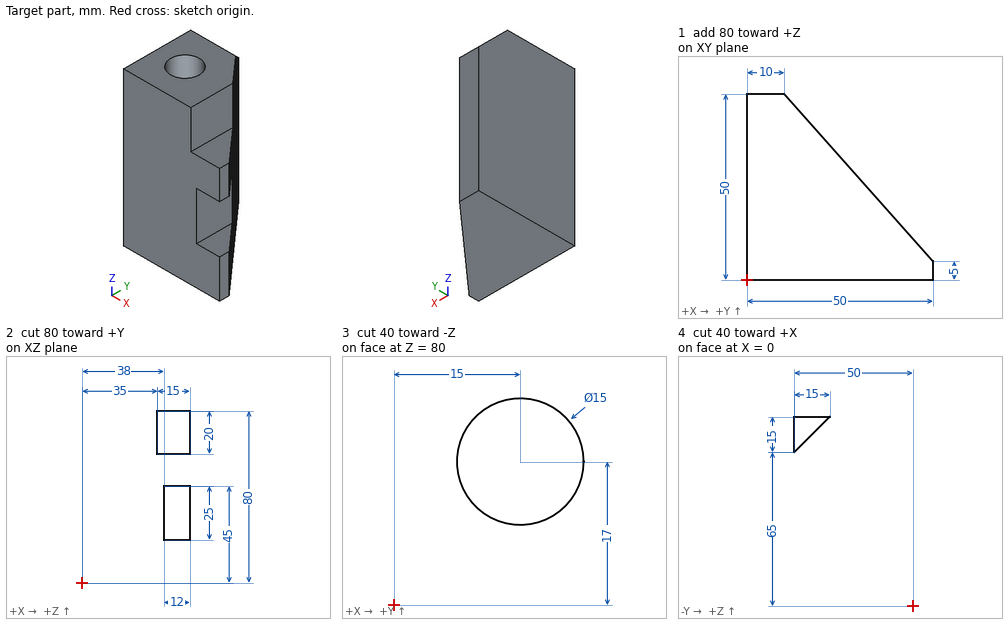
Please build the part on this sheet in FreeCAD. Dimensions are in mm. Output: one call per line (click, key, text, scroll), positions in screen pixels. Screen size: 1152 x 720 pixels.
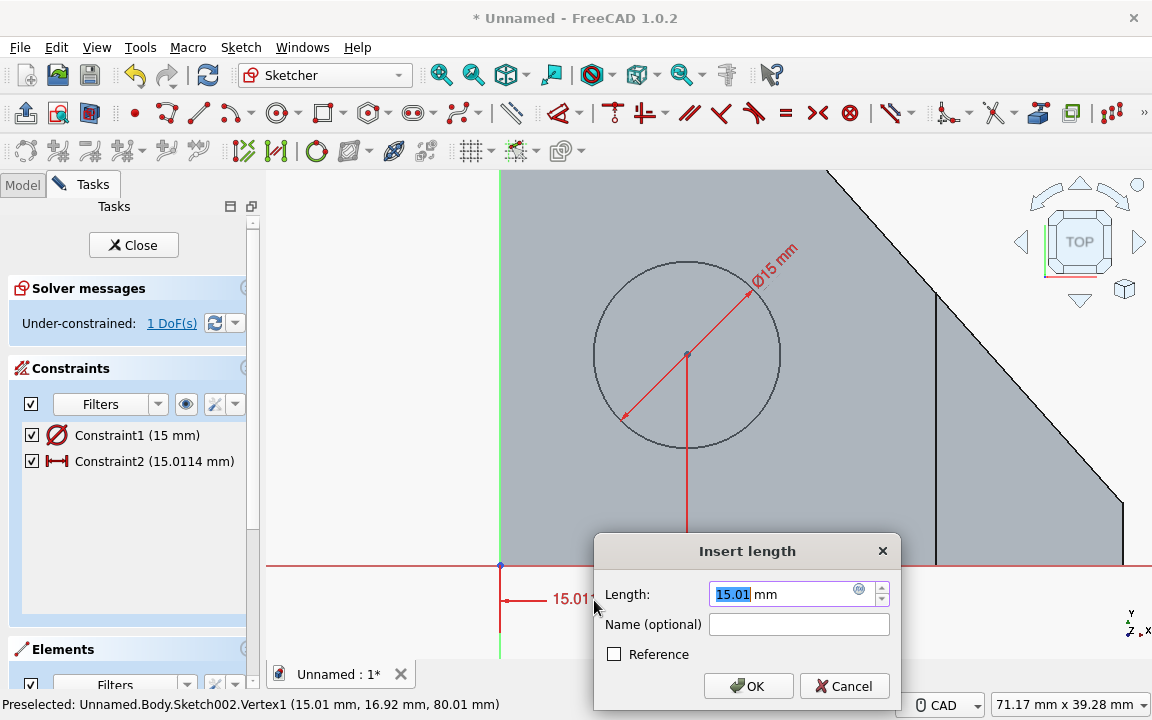
text(15)
key(Return)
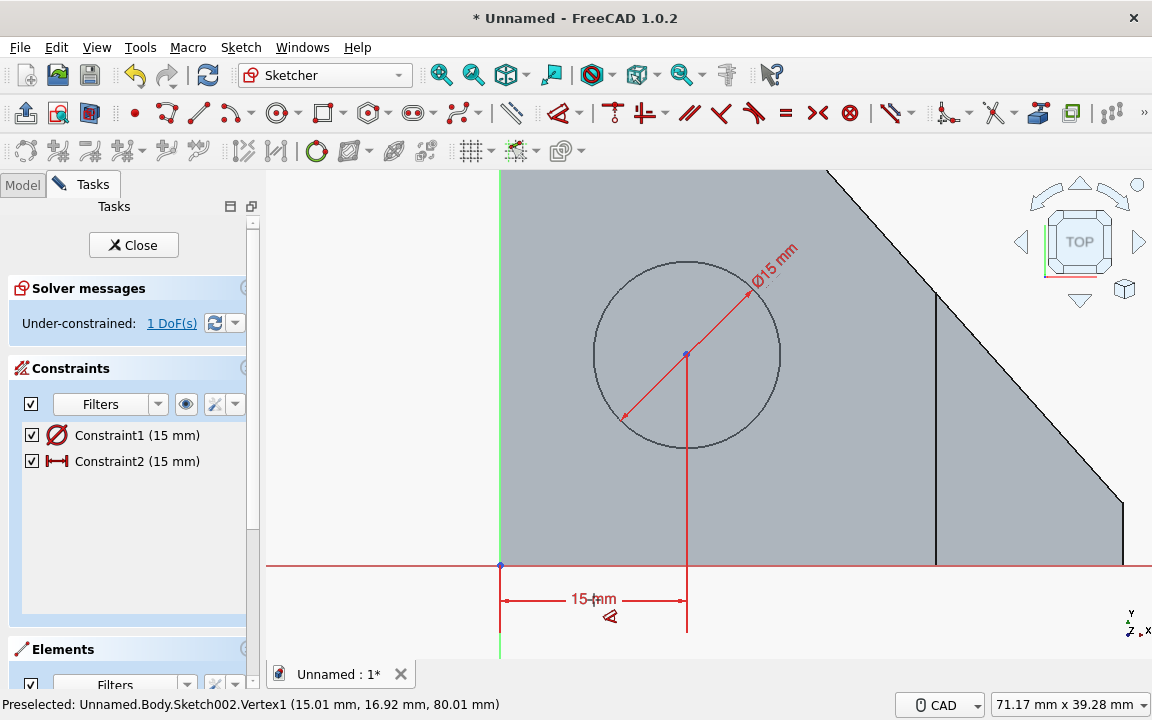
click(687, 355)
click(466, 460)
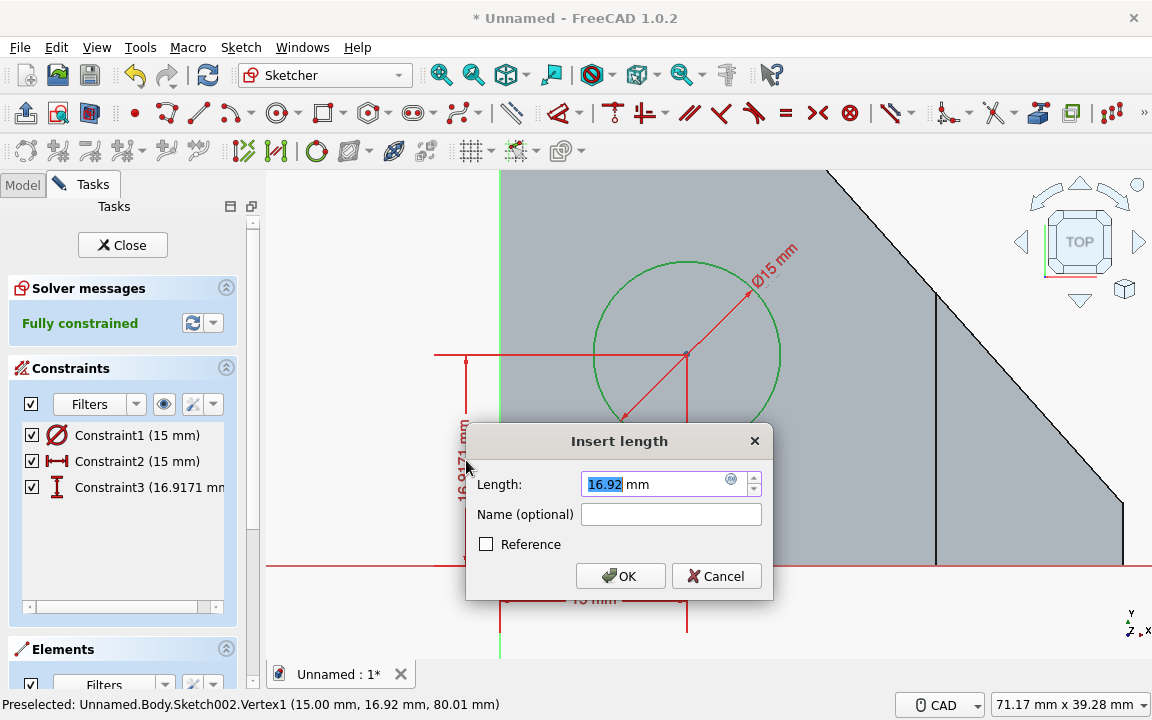
text(17)
key(Return)
key(Escape)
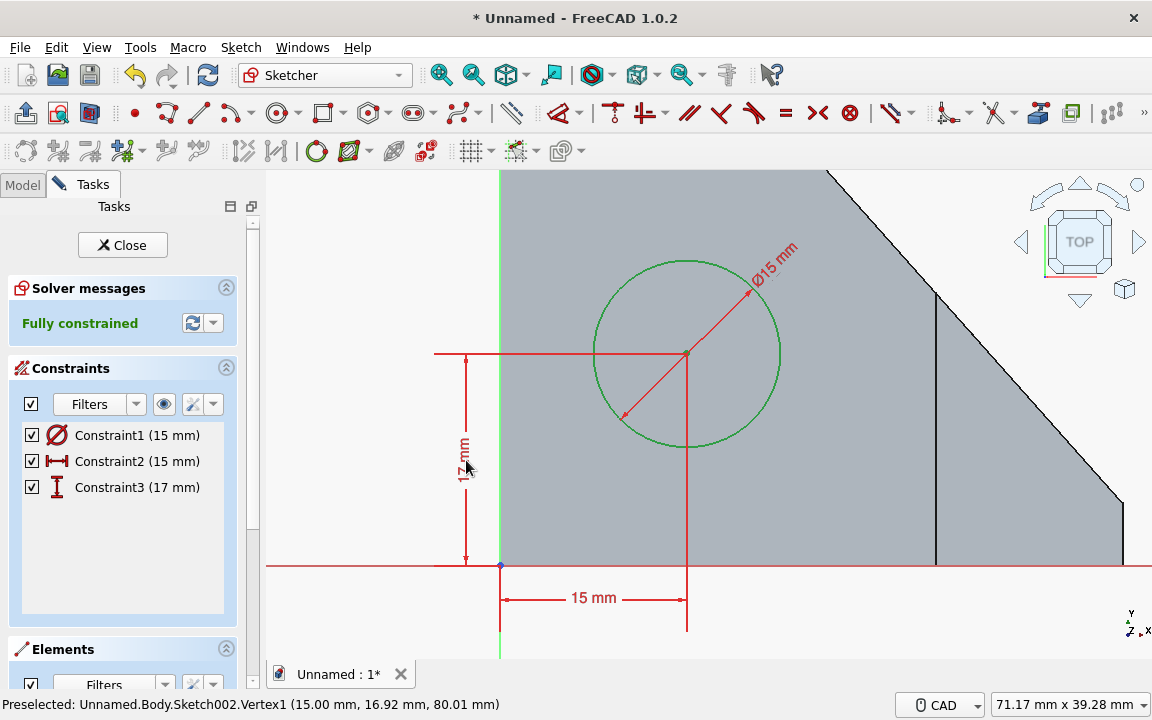
click(123, 245)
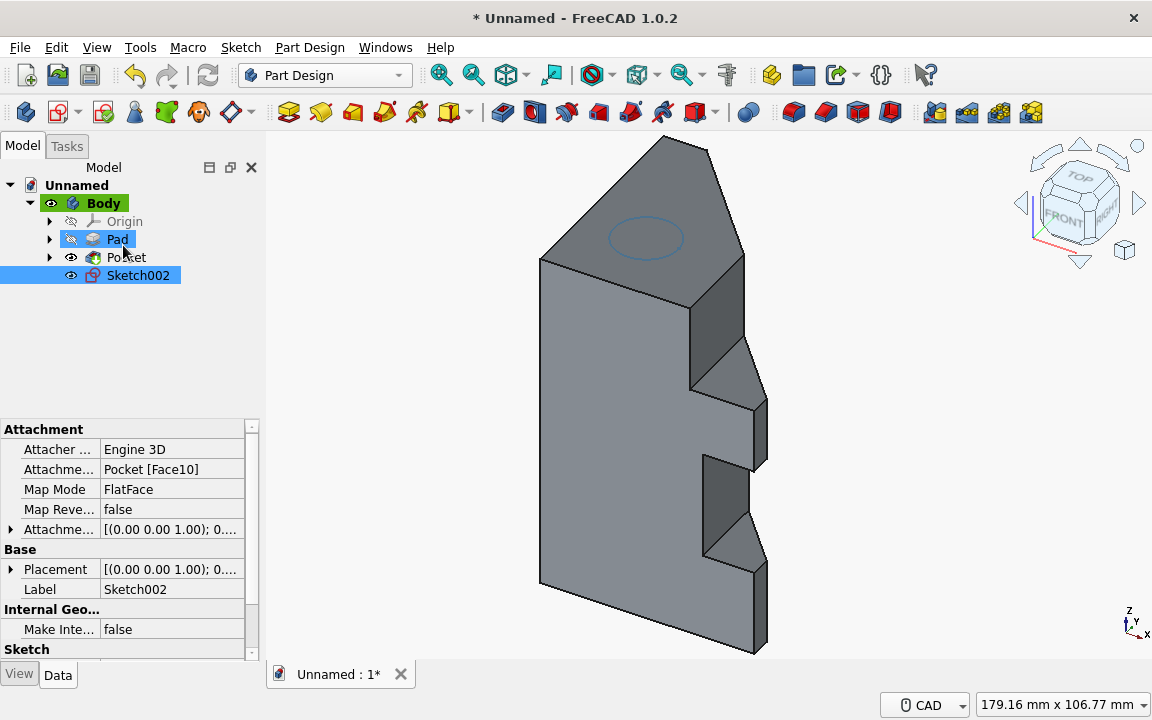
click(504, 112)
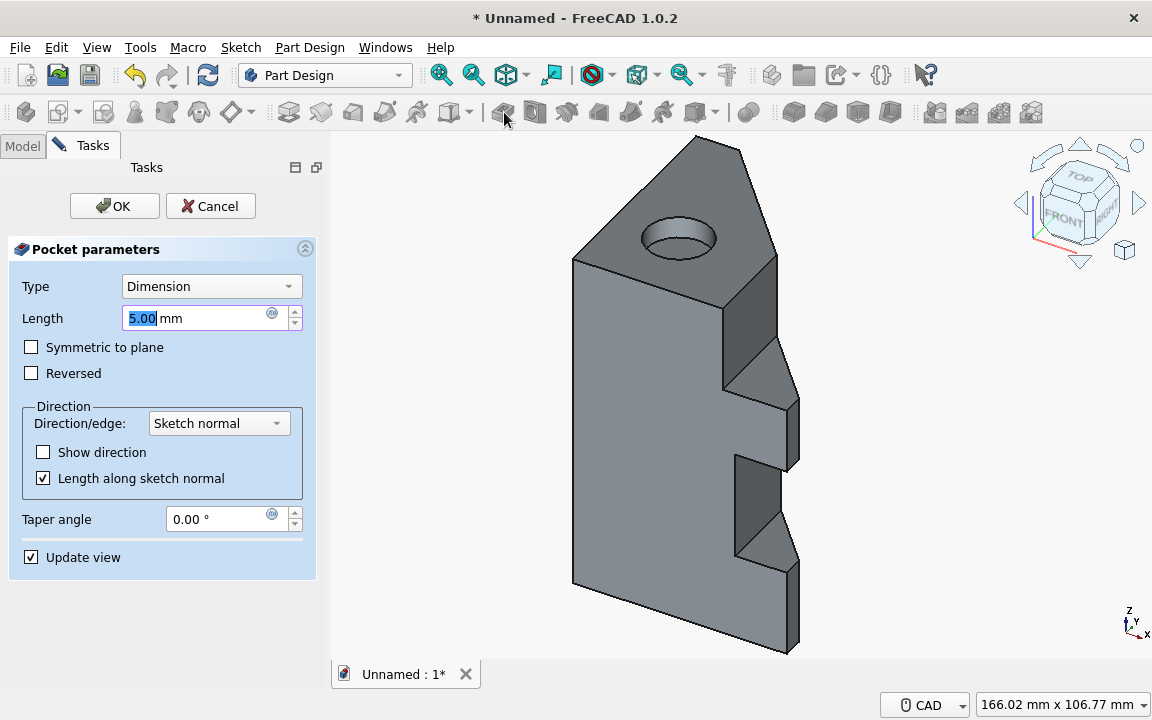
text(40)
key(Tab)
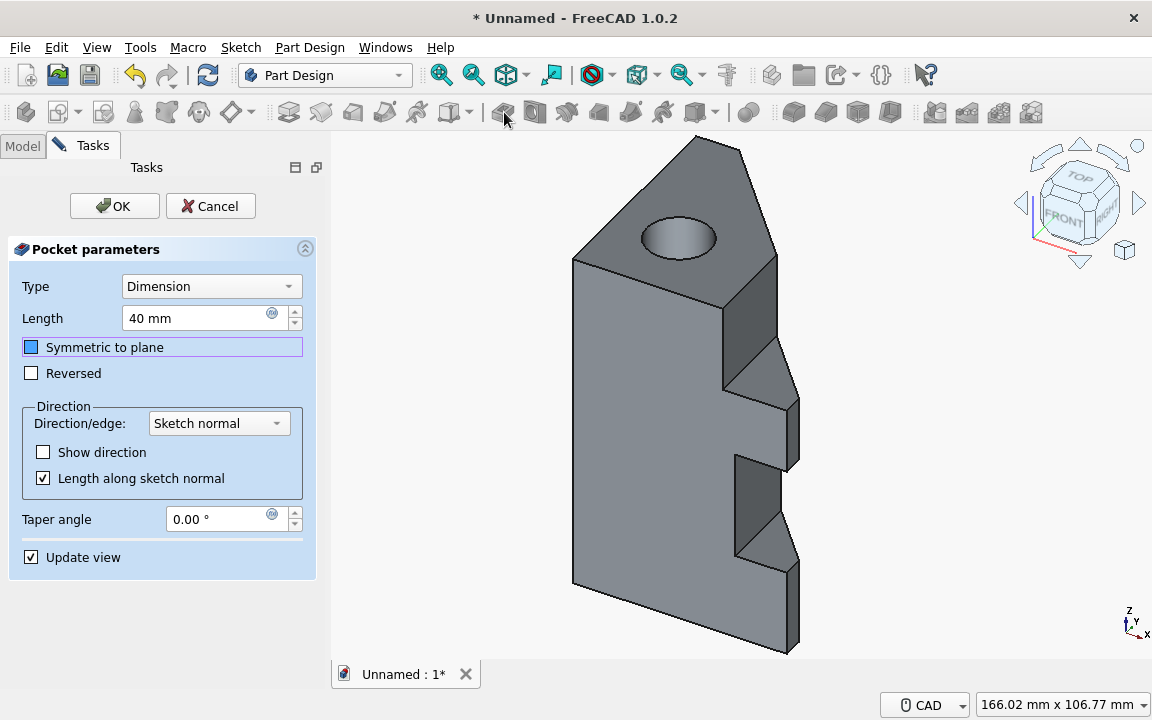
click(115, 206)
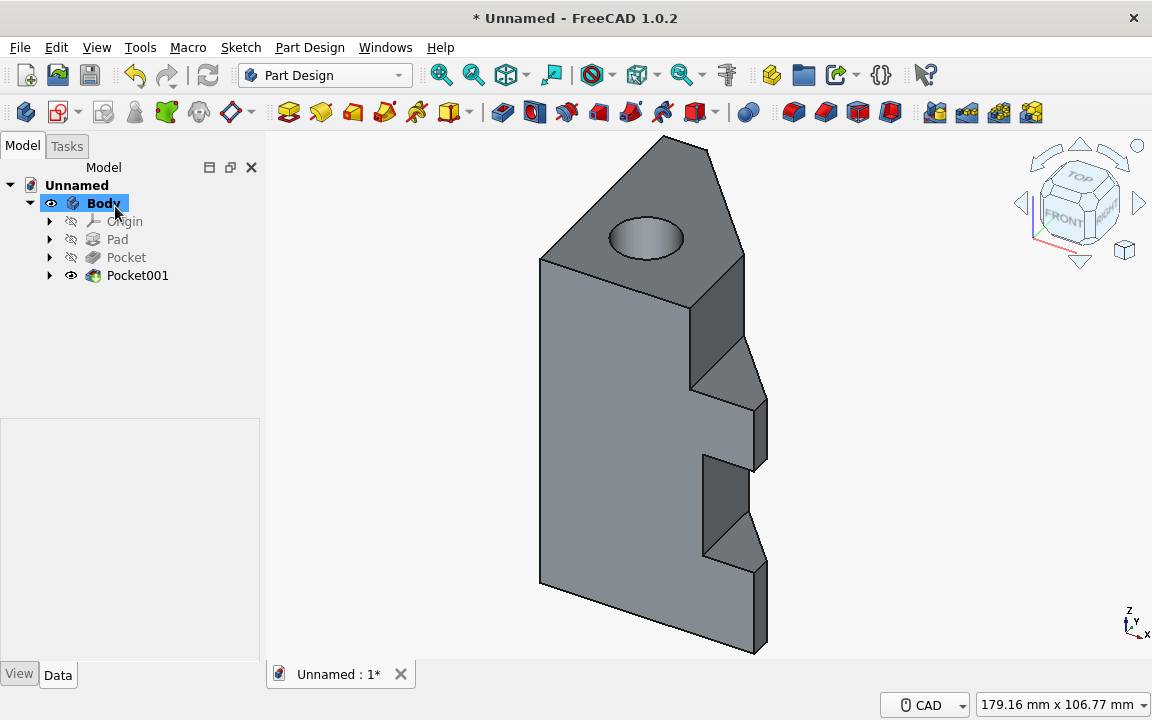
key(6)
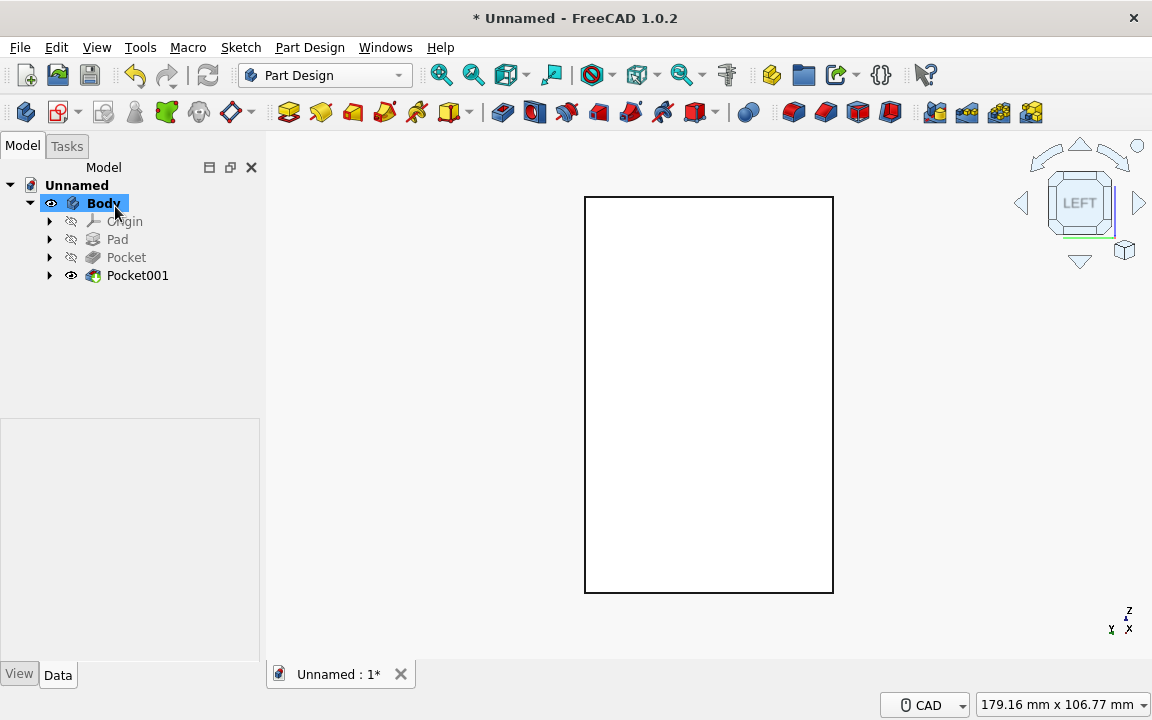
click(709, 337)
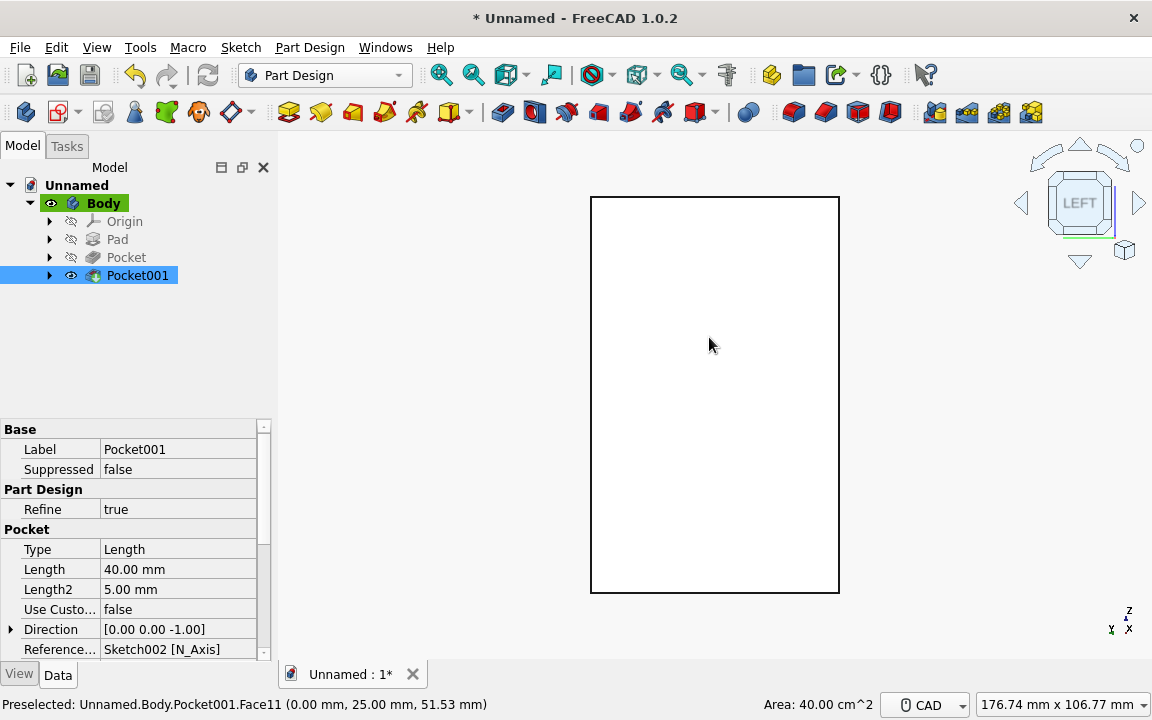
click(58, 112)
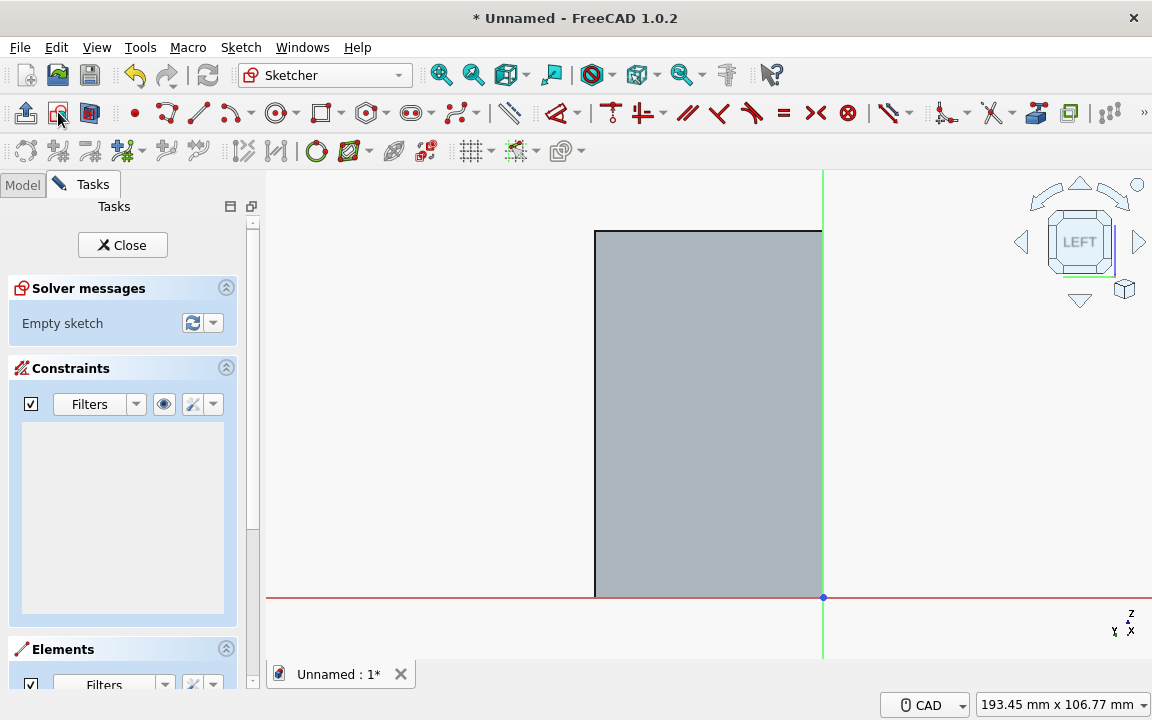
scroll(625, 217, up, 7)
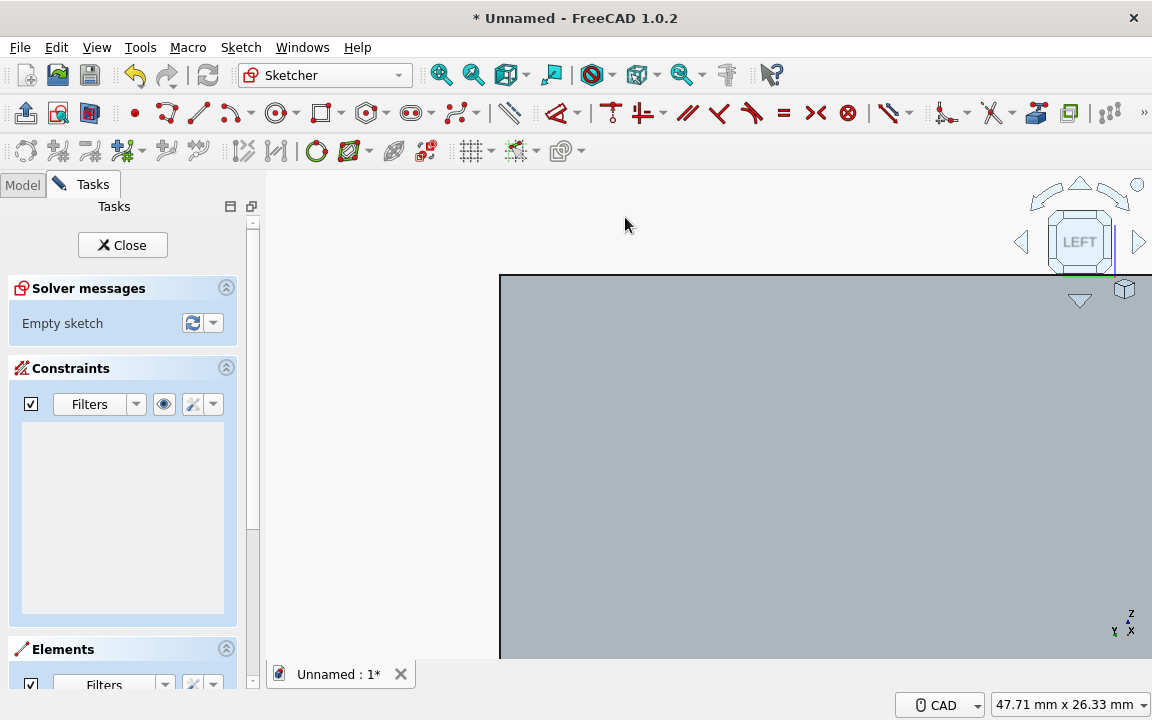
click(168, 114)